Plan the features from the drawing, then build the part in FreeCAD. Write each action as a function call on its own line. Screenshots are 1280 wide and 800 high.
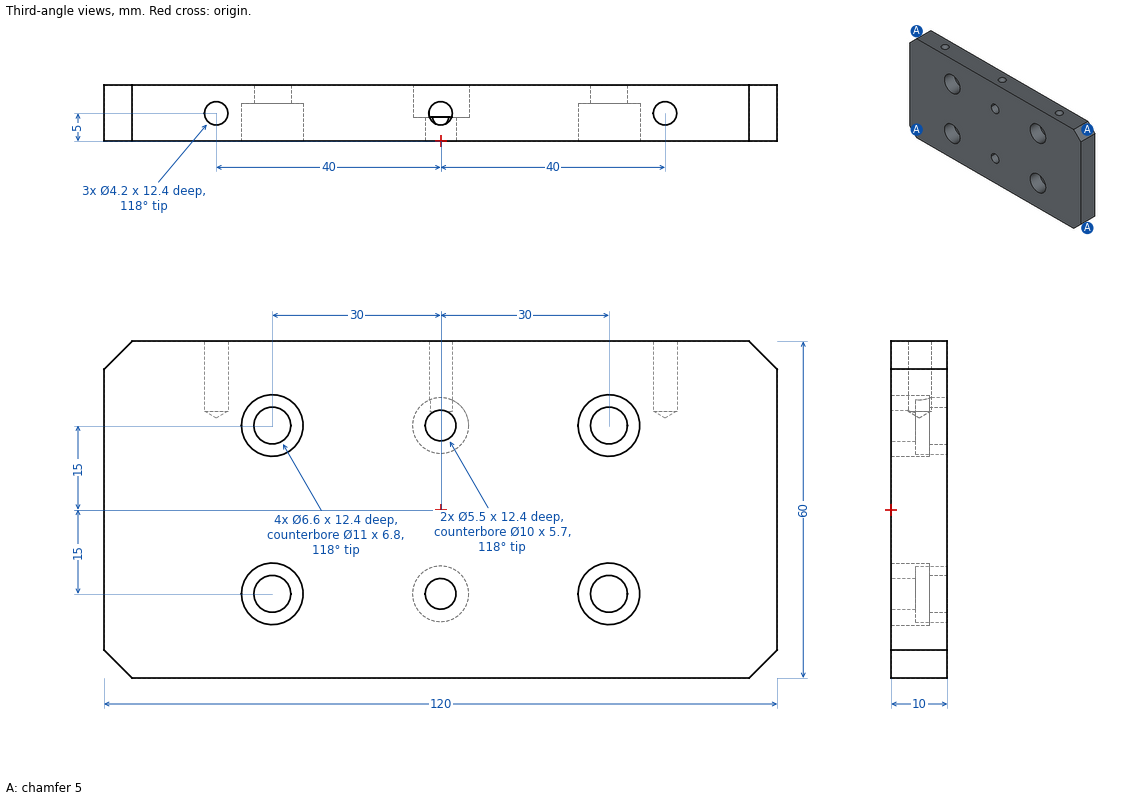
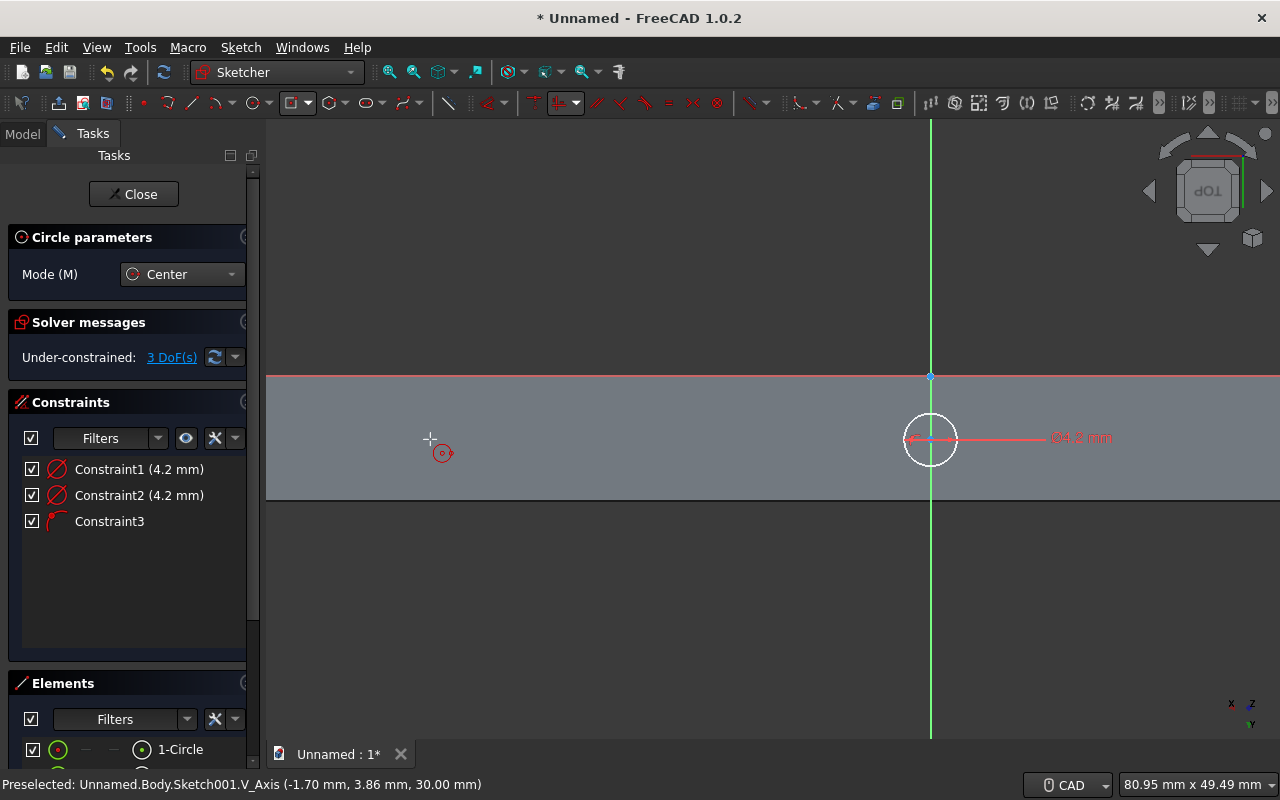
click(429, 439)
move(448, 420)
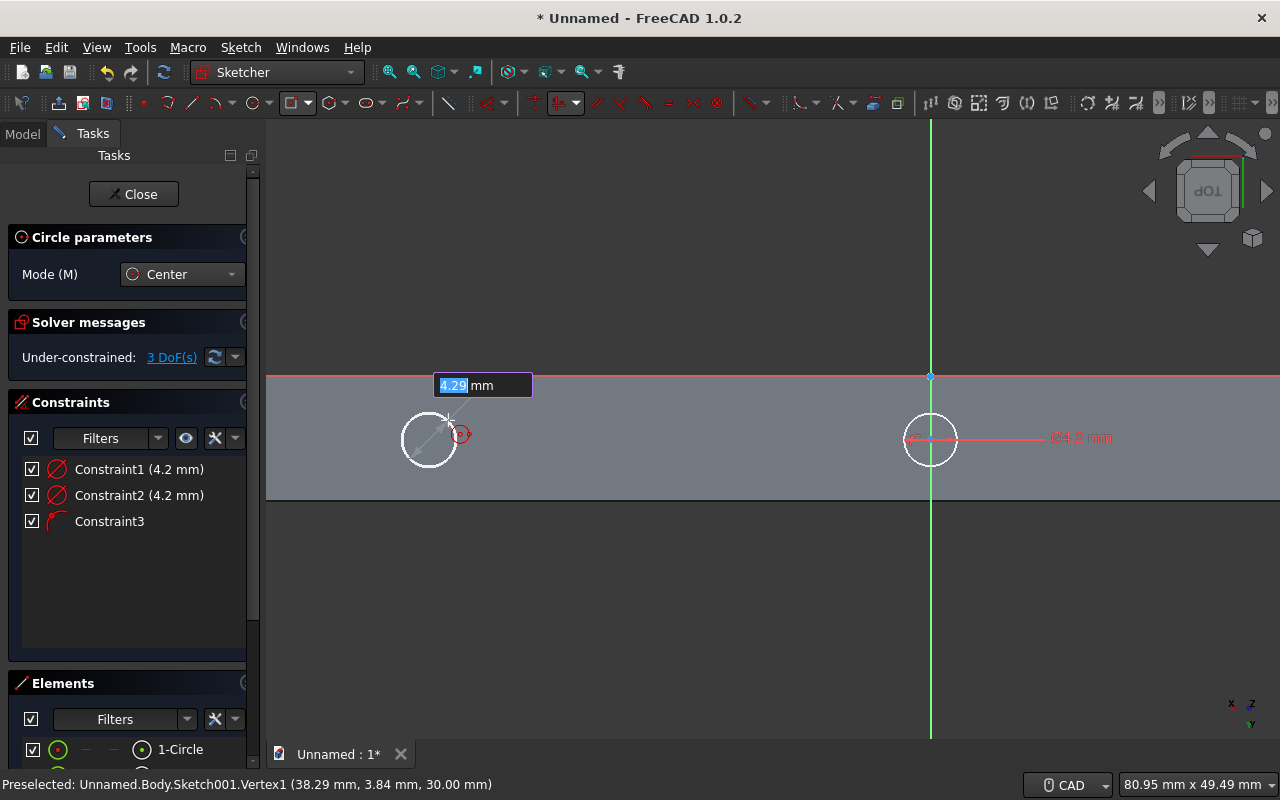
text(4.2)
key(Return)
key(Escape)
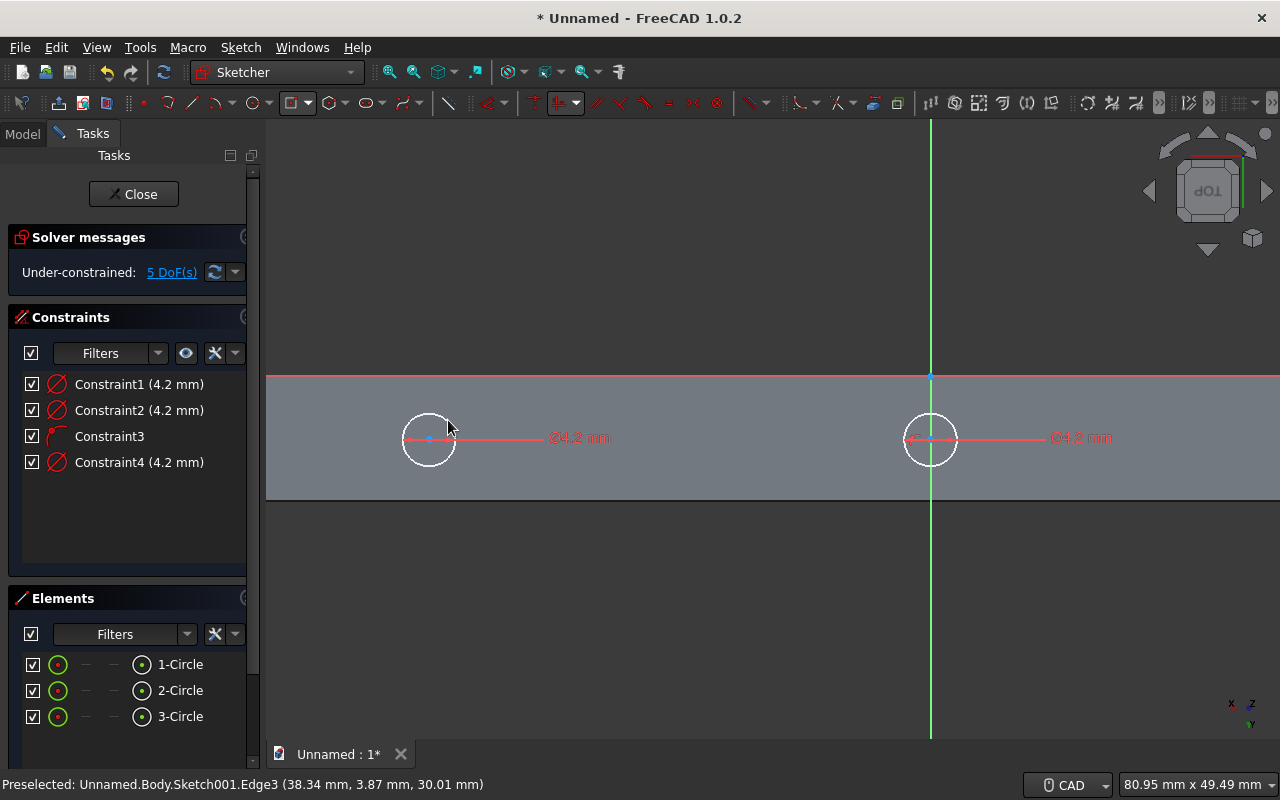
scroll(430, 439, down, 3)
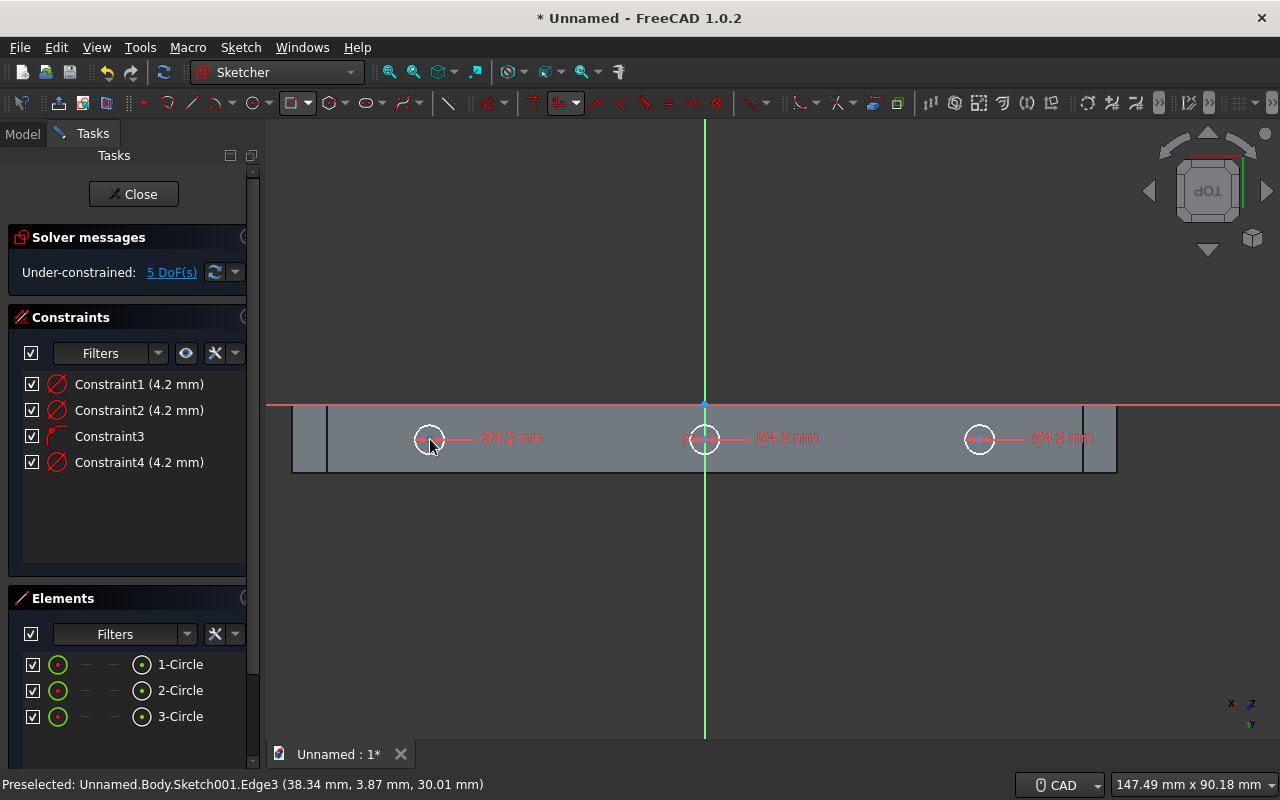
click(980, 440)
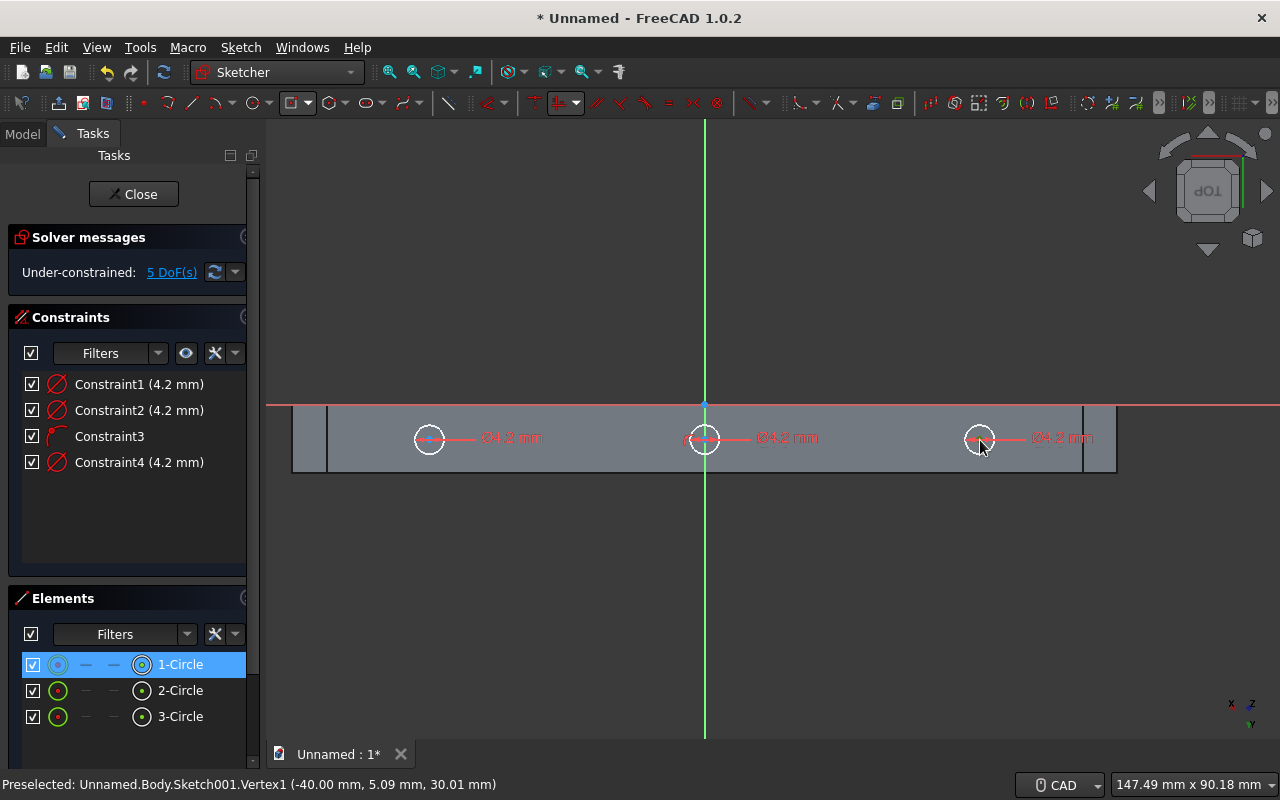
click(705, 440)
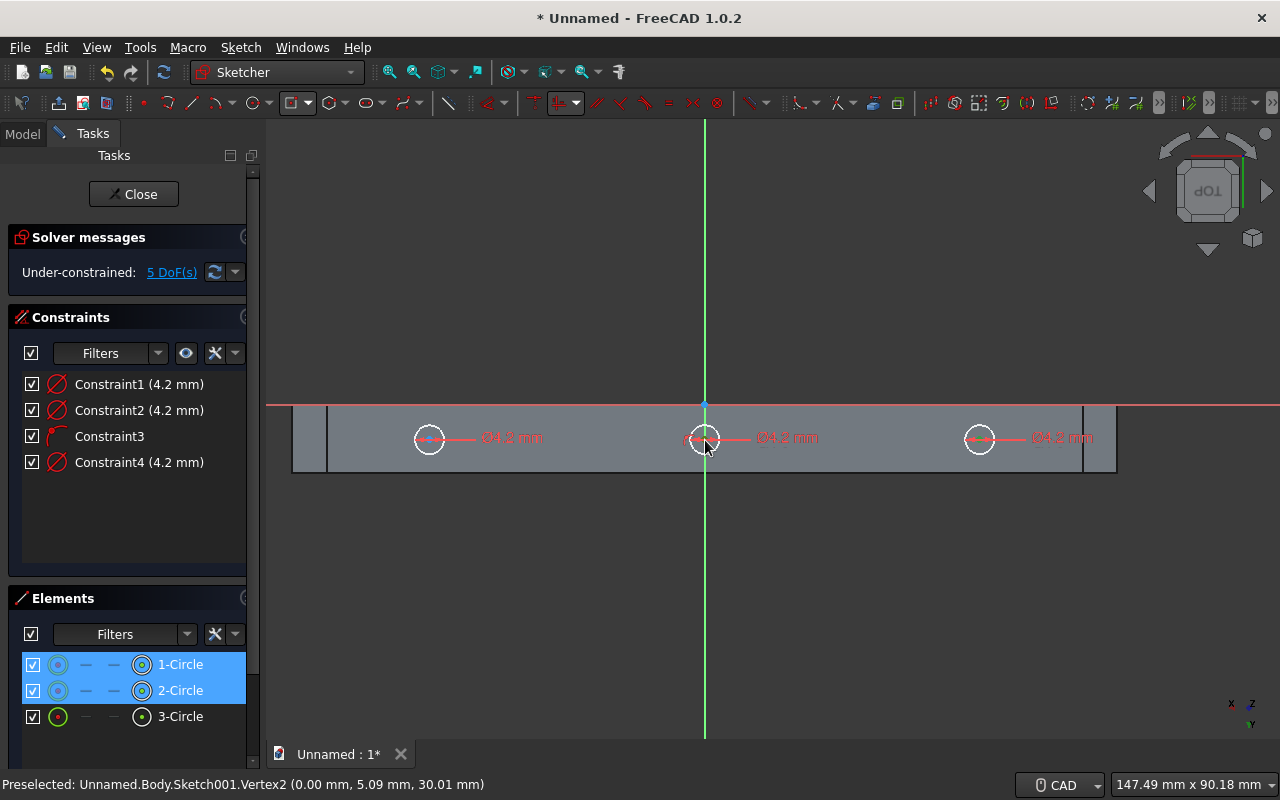
key(h)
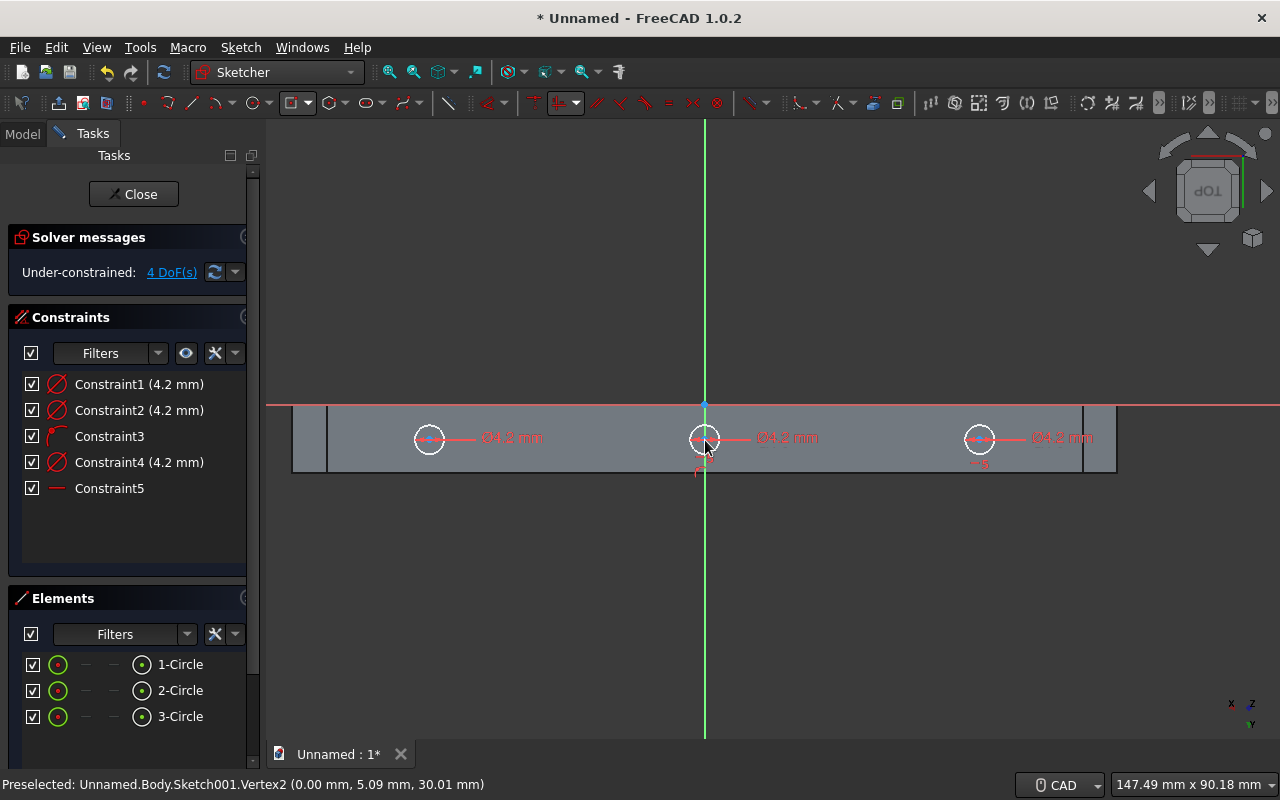
click(705, 440)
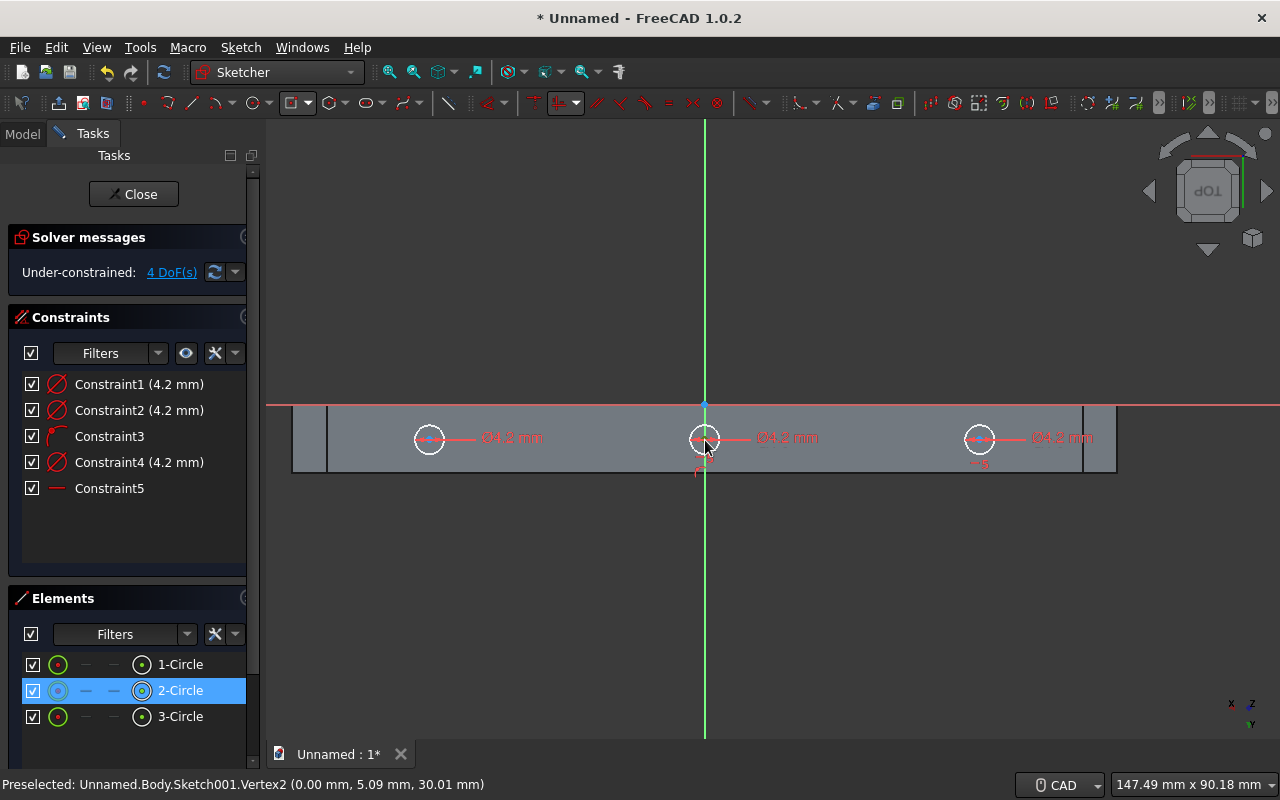
click(430, 440)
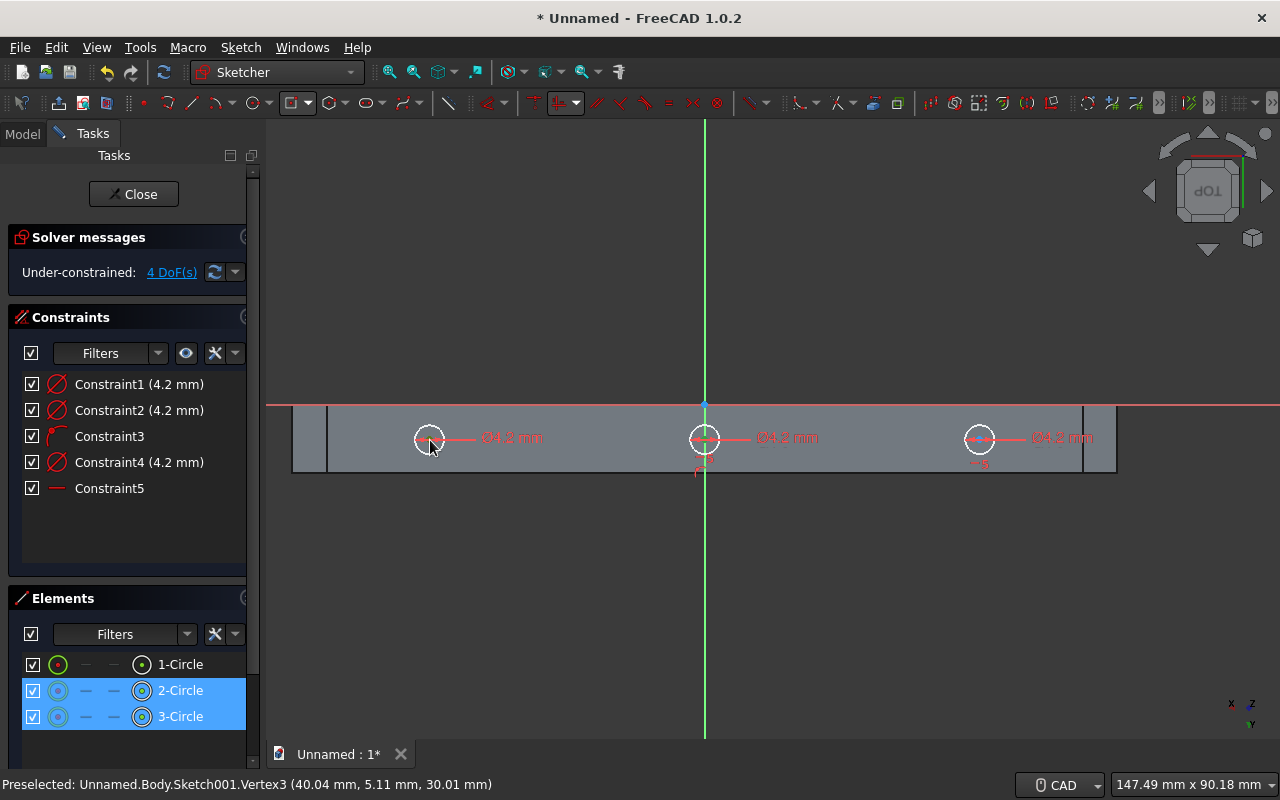
key(h)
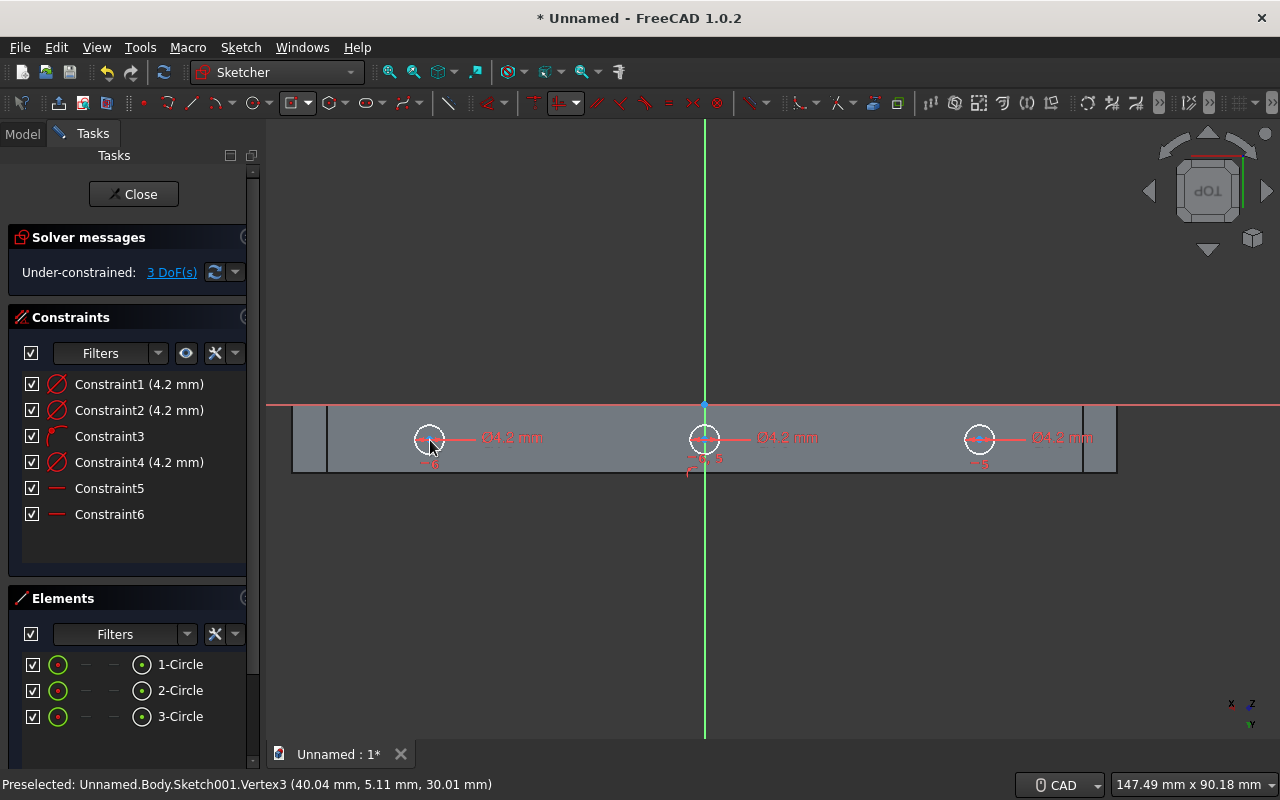
click(980, 440)